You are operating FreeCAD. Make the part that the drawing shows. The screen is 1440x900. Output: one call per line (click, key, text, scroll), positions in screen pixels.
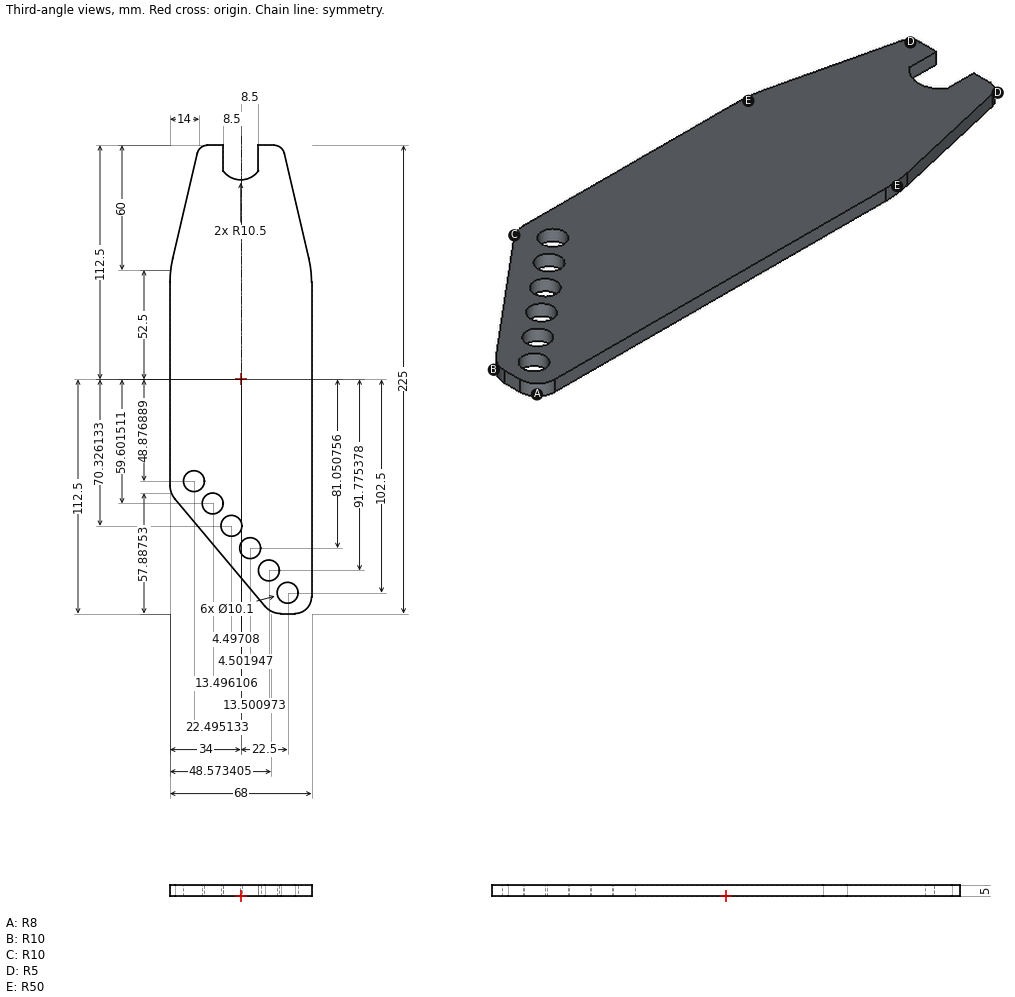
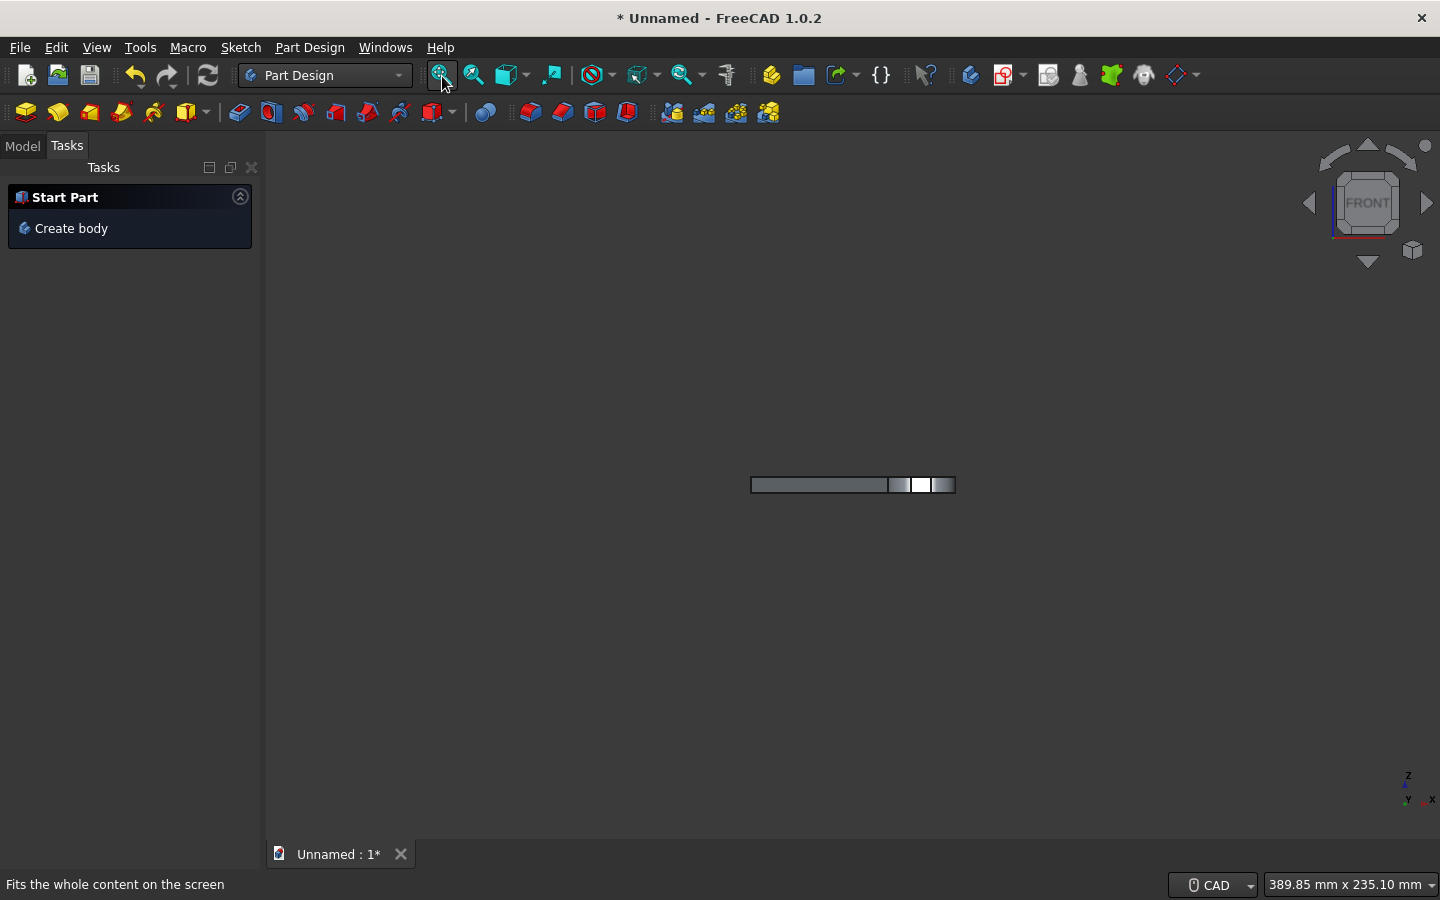
key(v)
key(f)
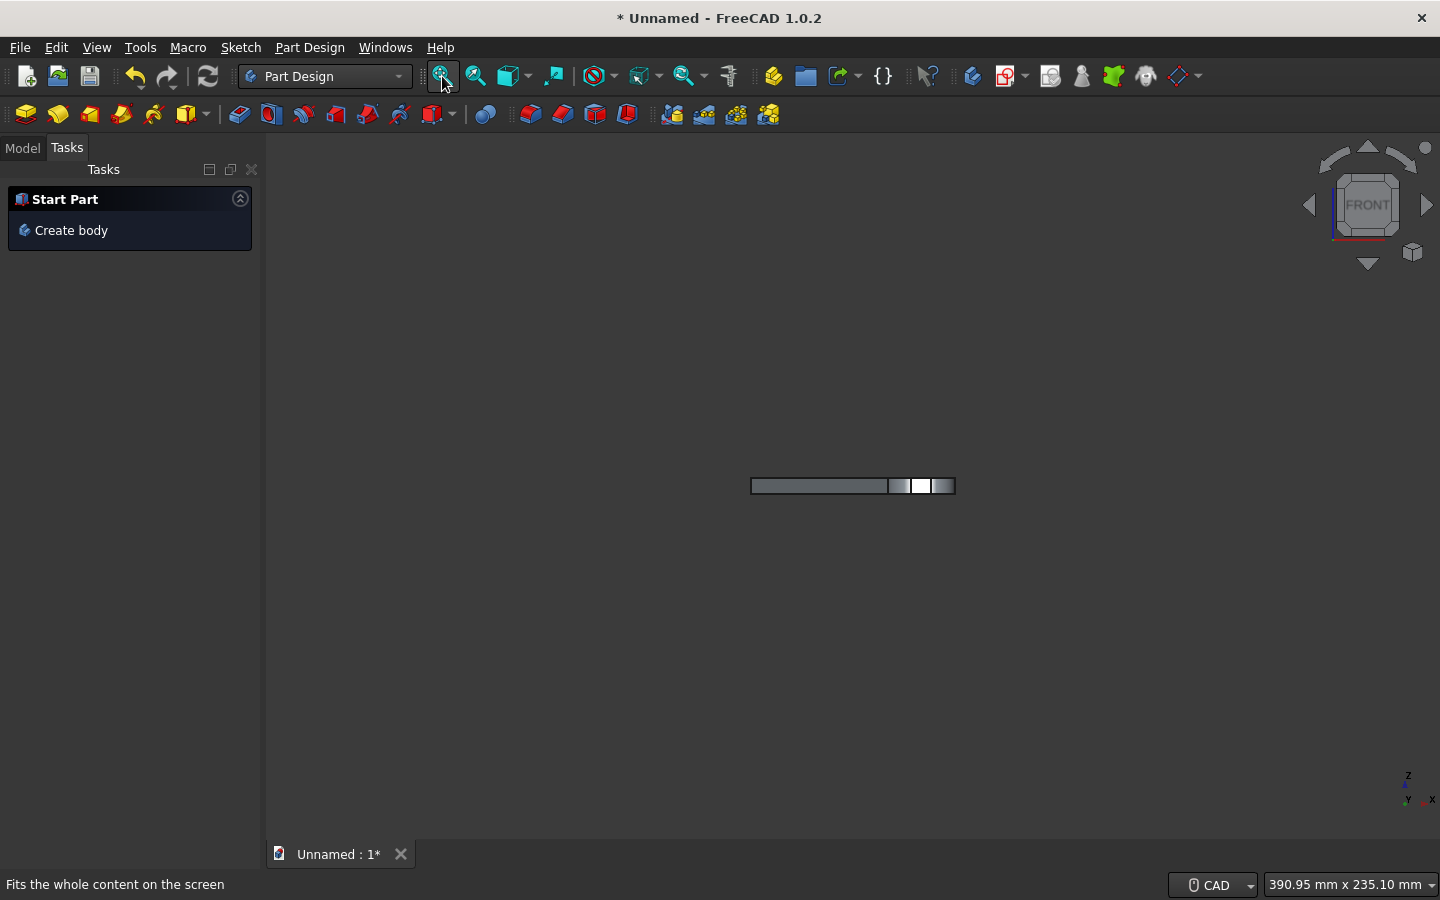
scroll(751, 485, up, 5)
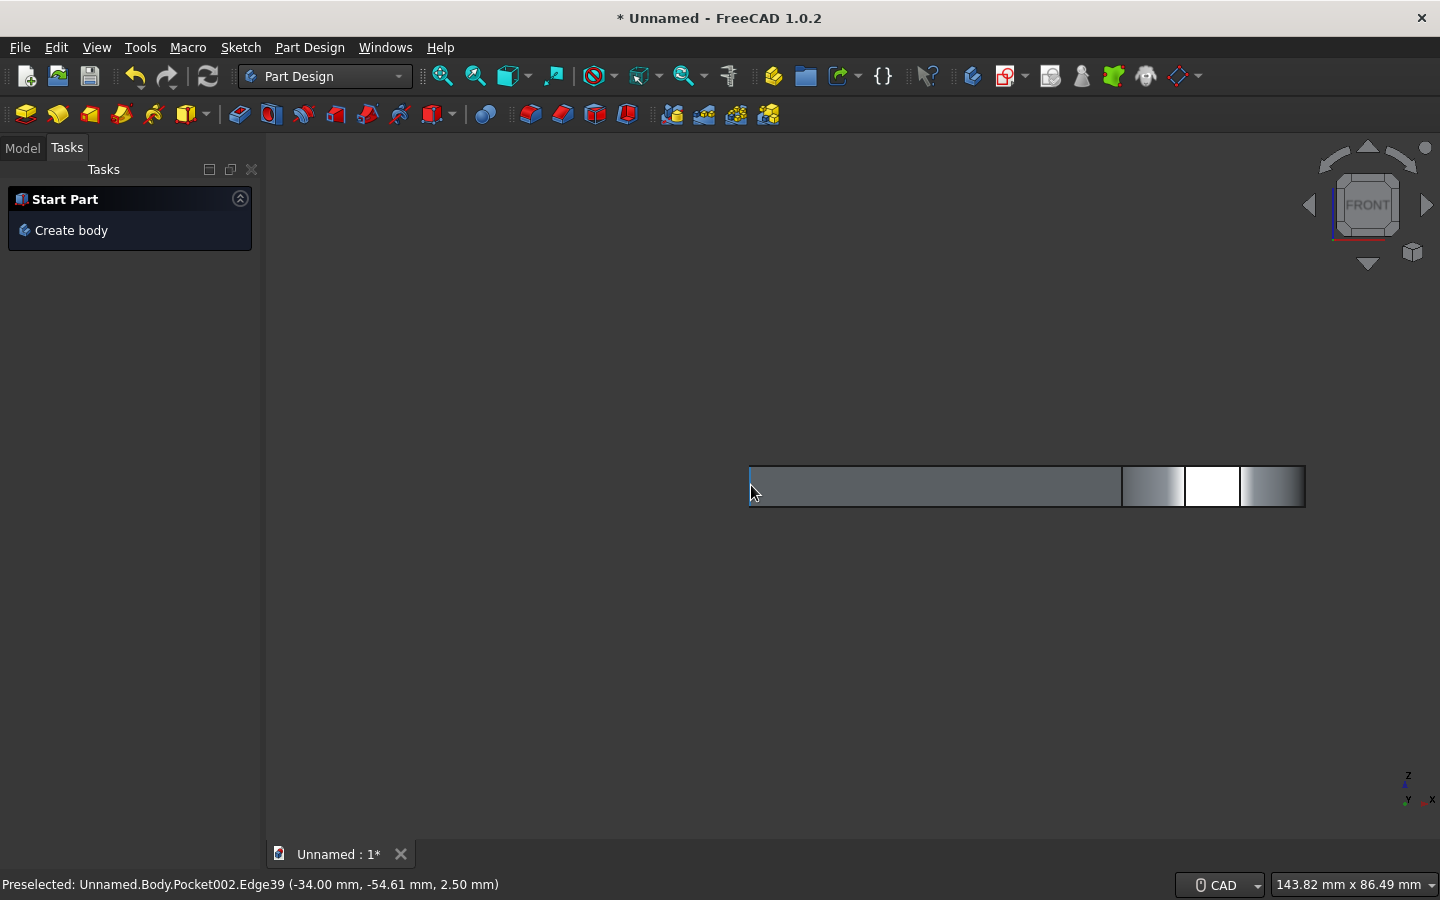
key(v)
key(f)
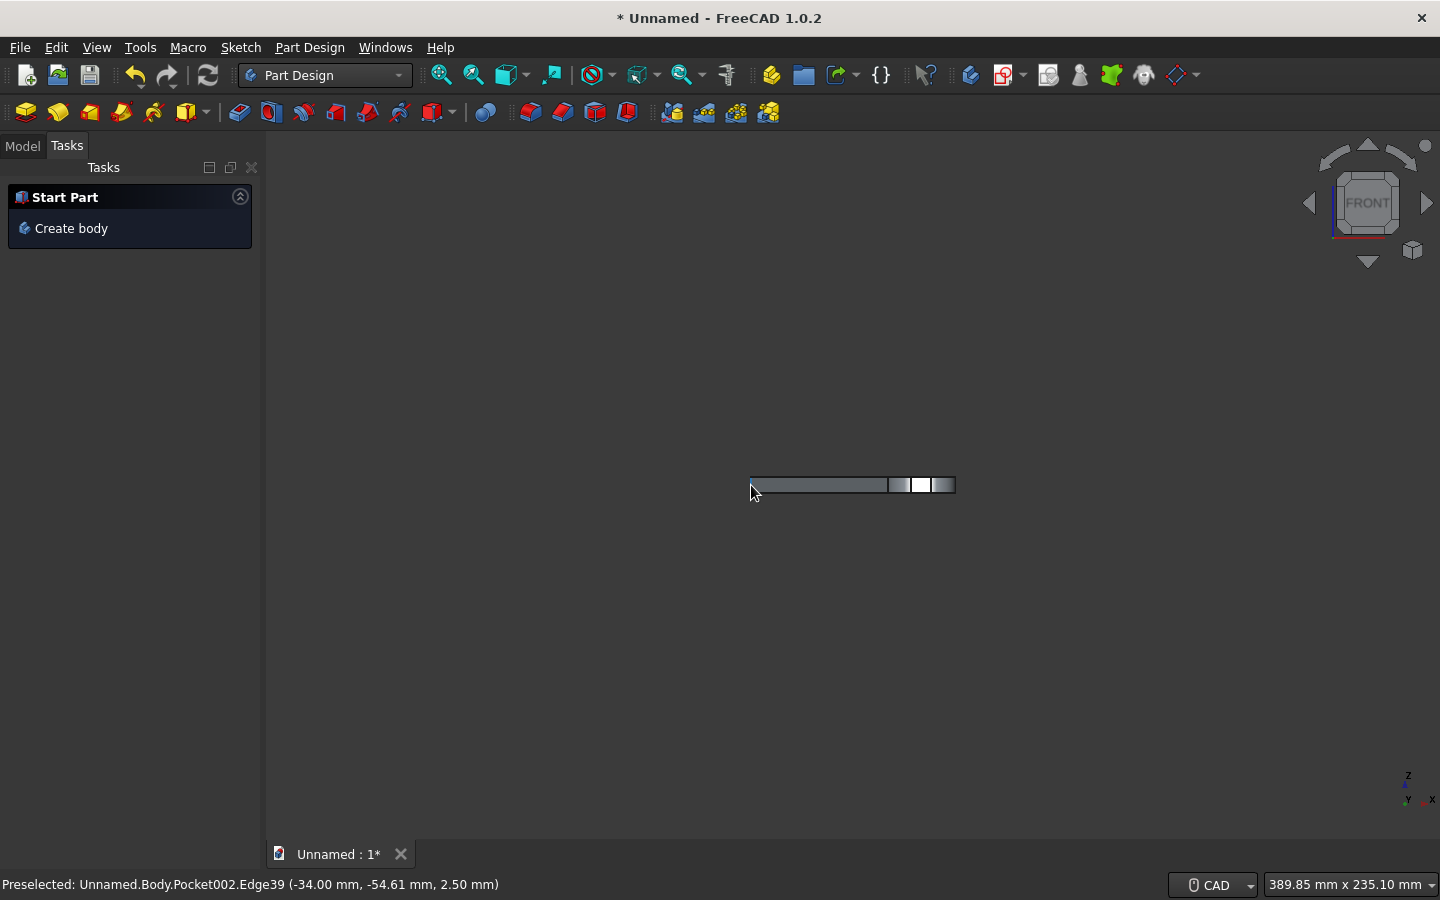
key(3)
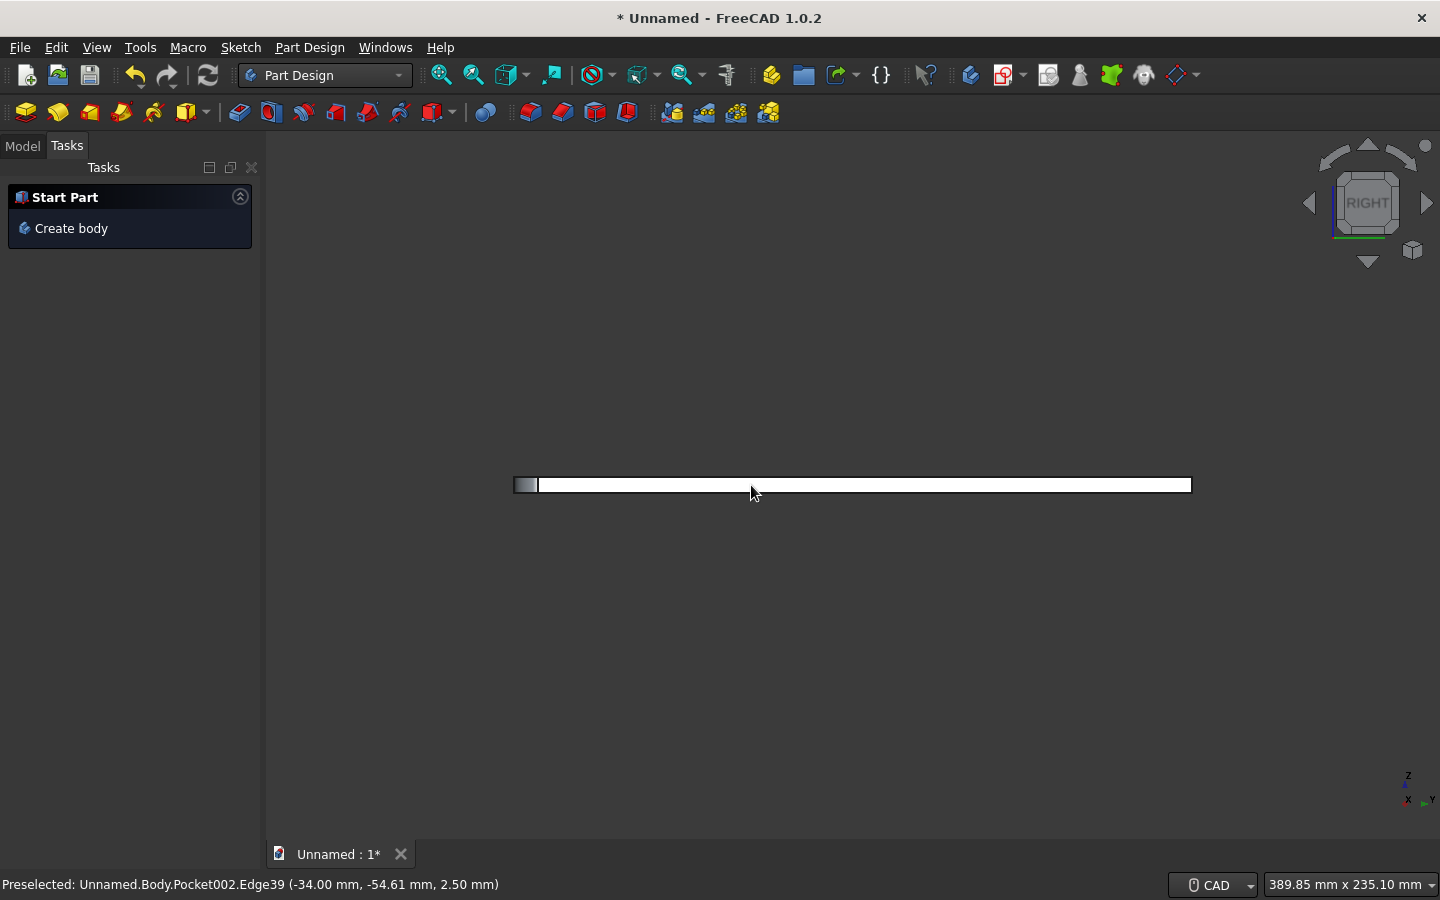
scroll(689, 484, up, 5)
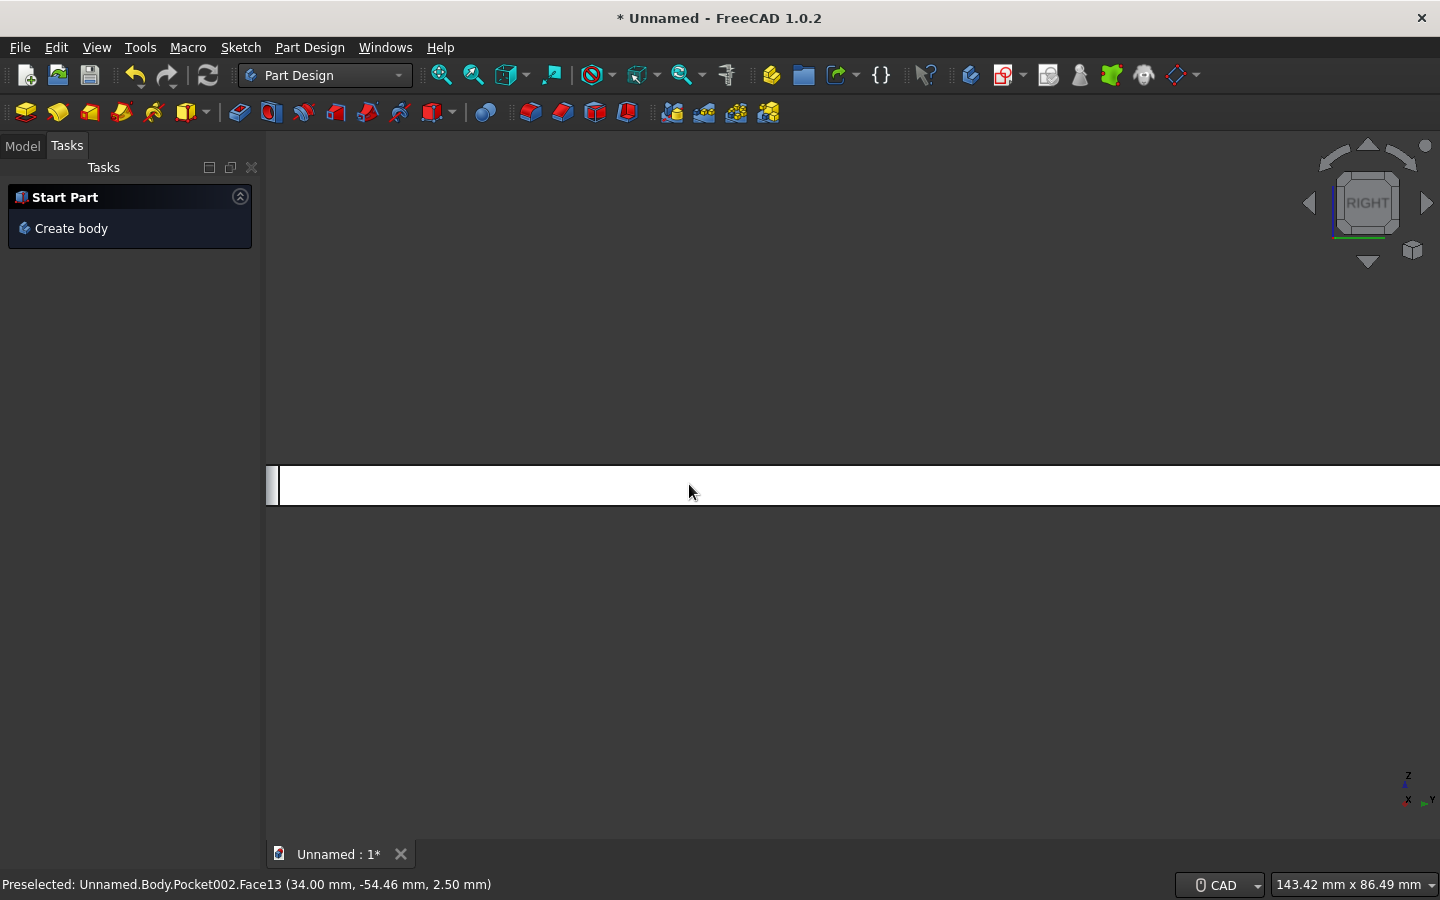
key(v)
key(f)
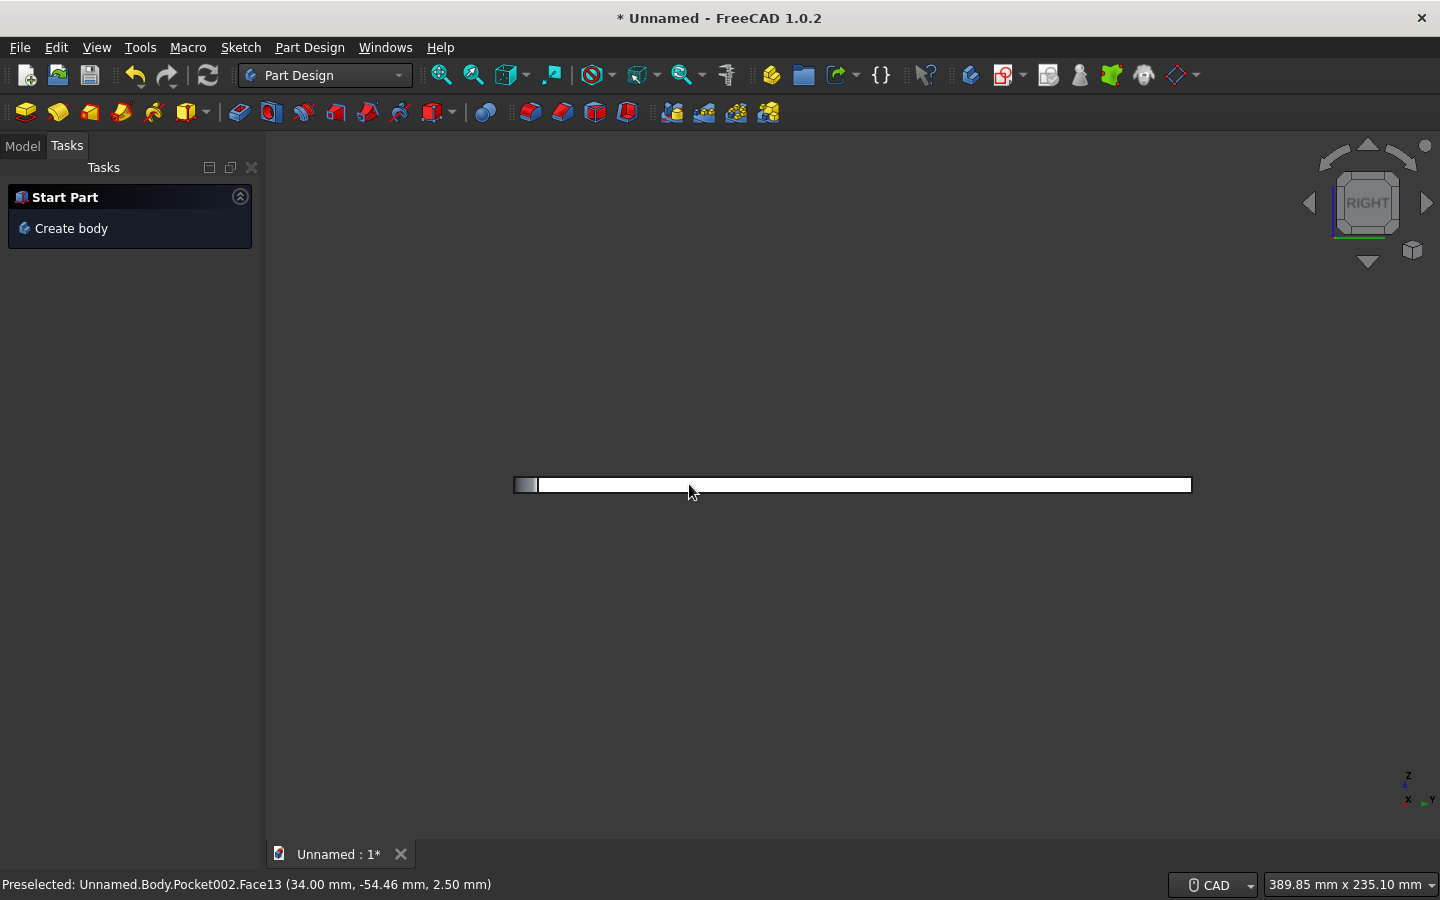
key(5)